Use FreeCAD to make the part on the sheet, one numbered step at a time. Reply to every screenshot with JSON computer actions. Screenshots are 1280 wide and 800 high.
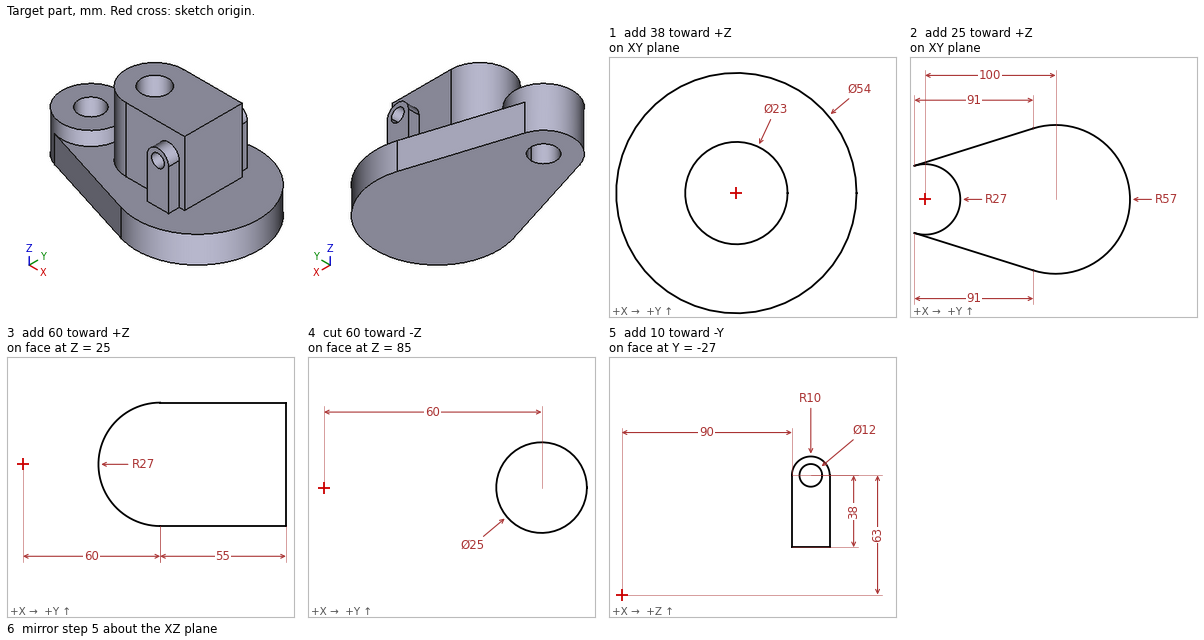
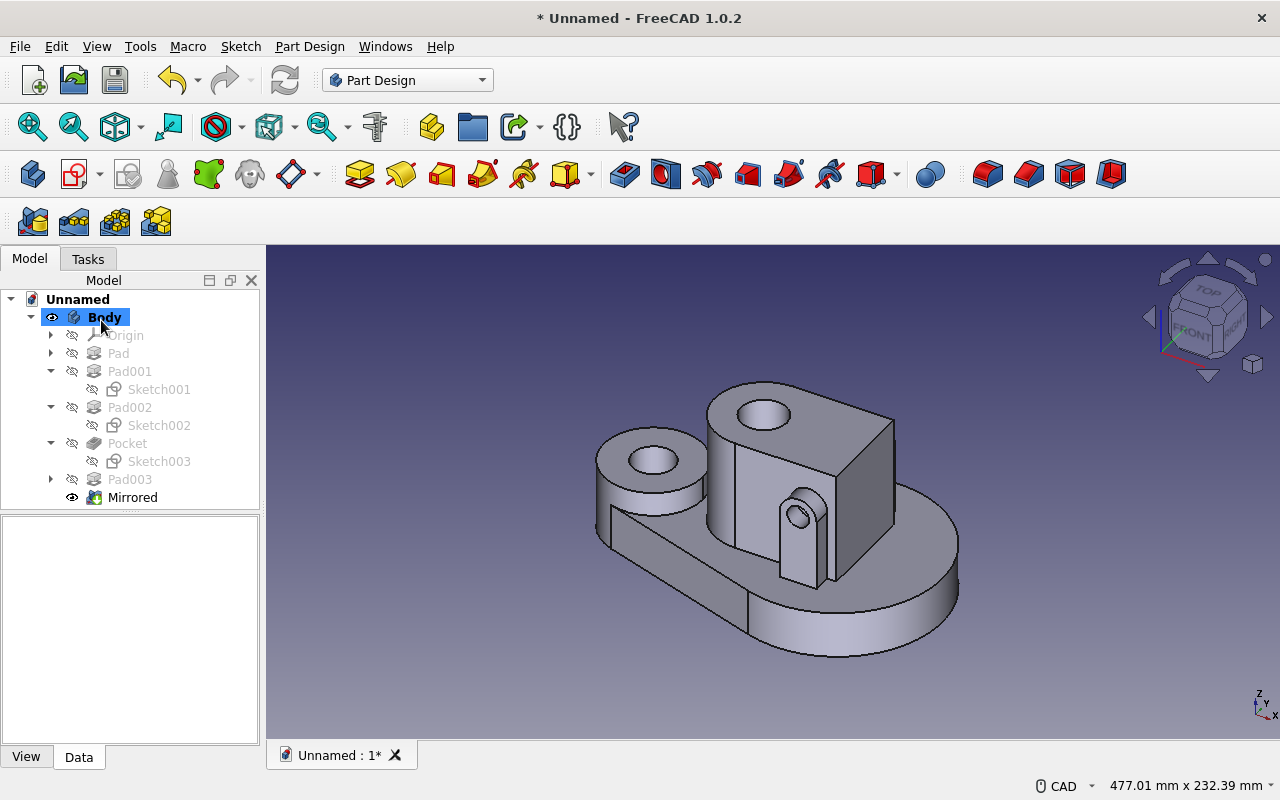
{"action": "key", "text": "0"}